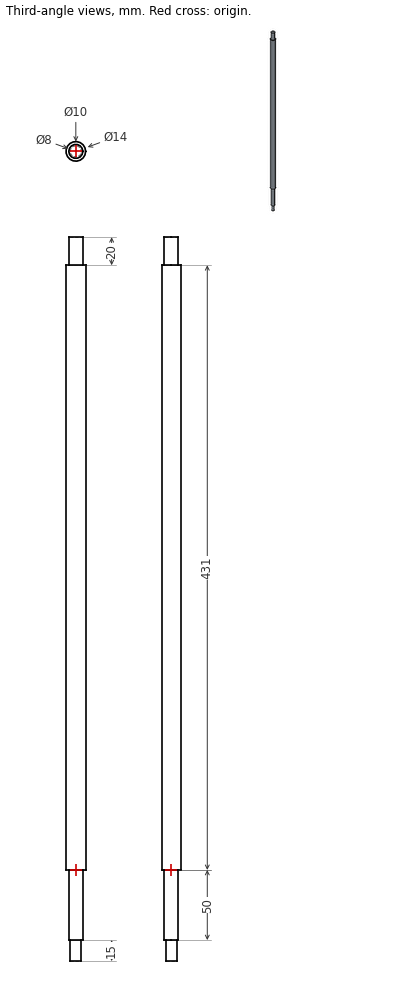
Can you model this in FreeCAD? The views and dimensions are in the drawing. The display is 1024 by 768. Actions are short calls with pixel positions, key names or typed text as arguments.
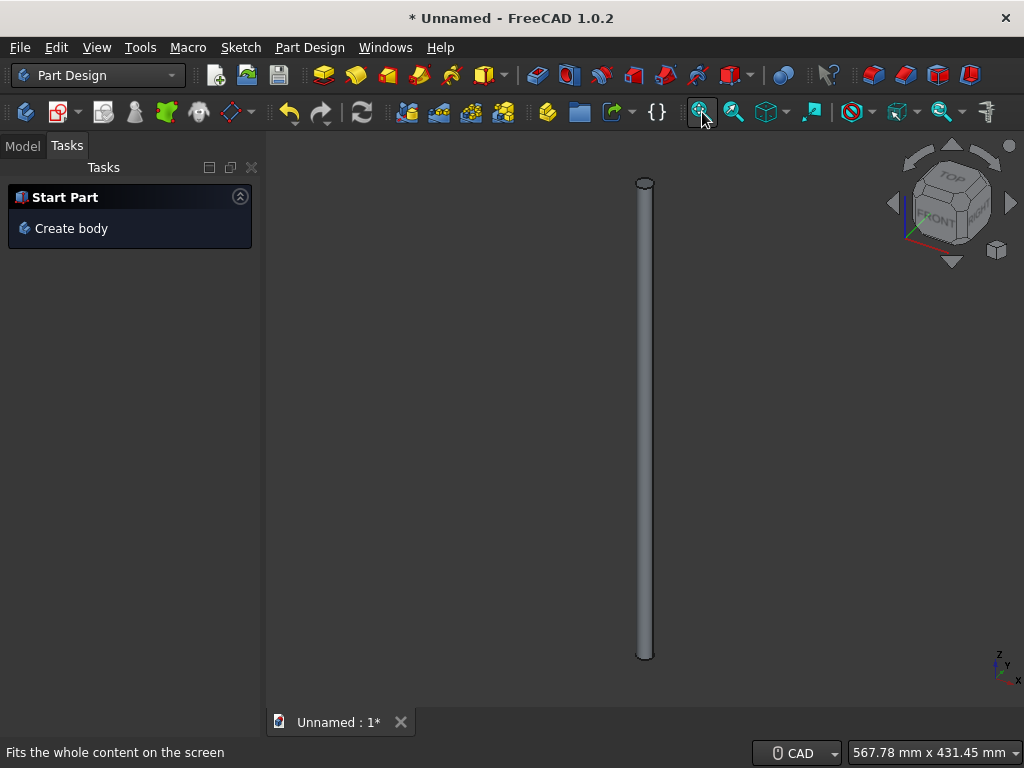
key(0)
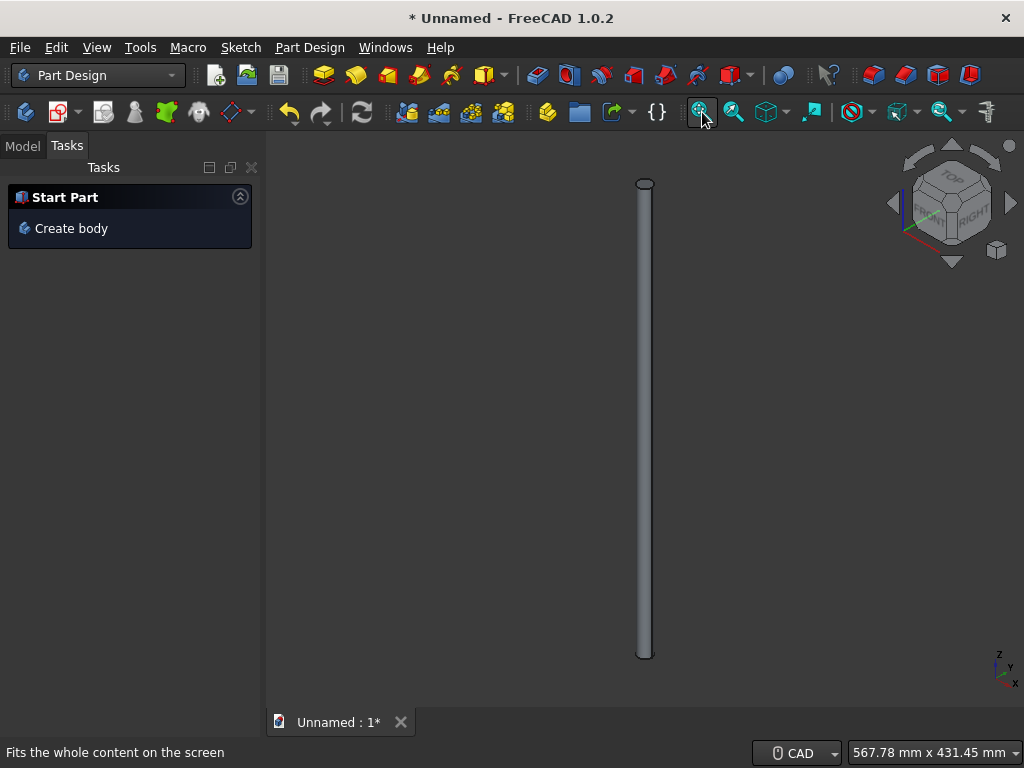
key(2)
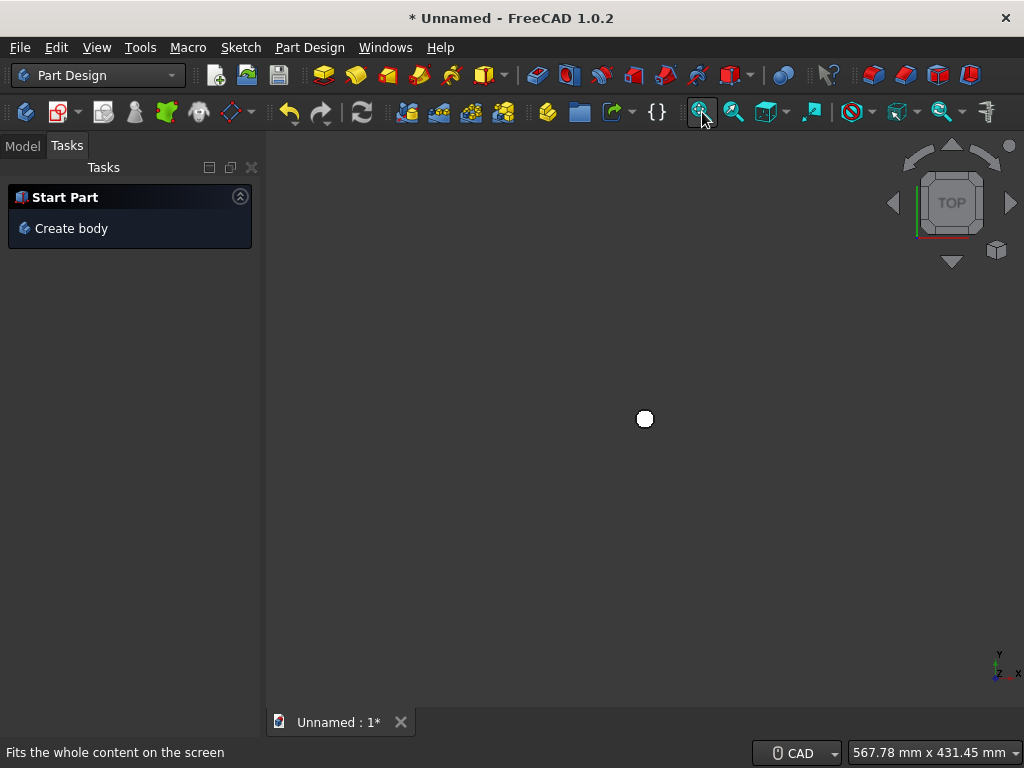
click(702, 112)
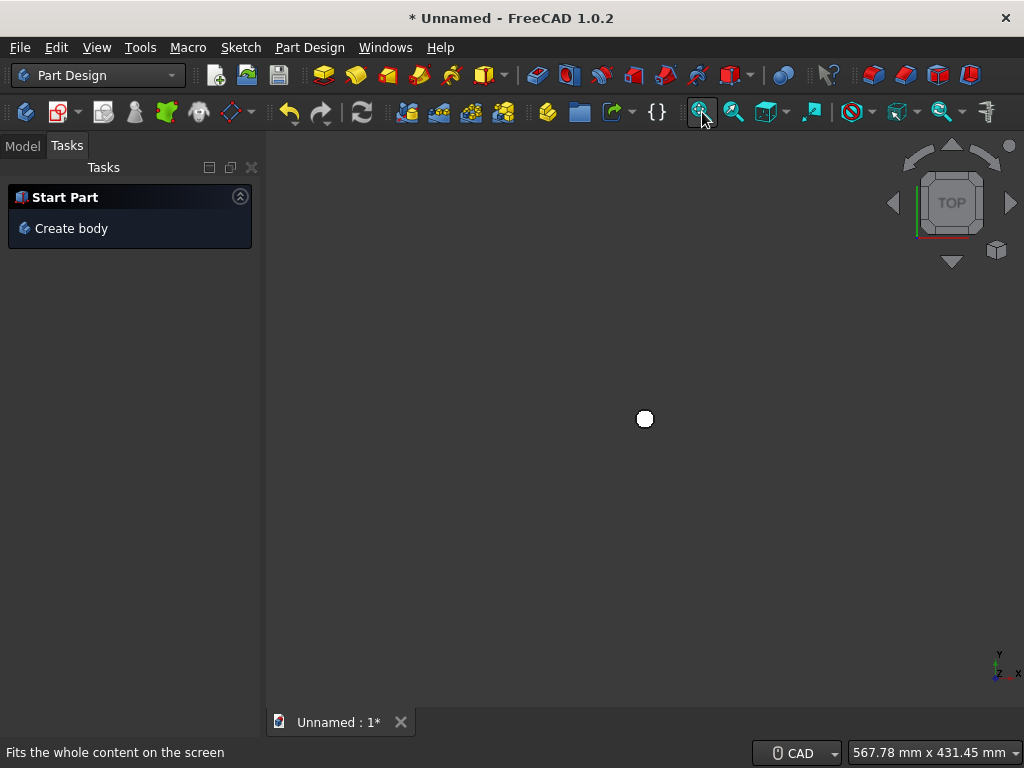
click(645, 418)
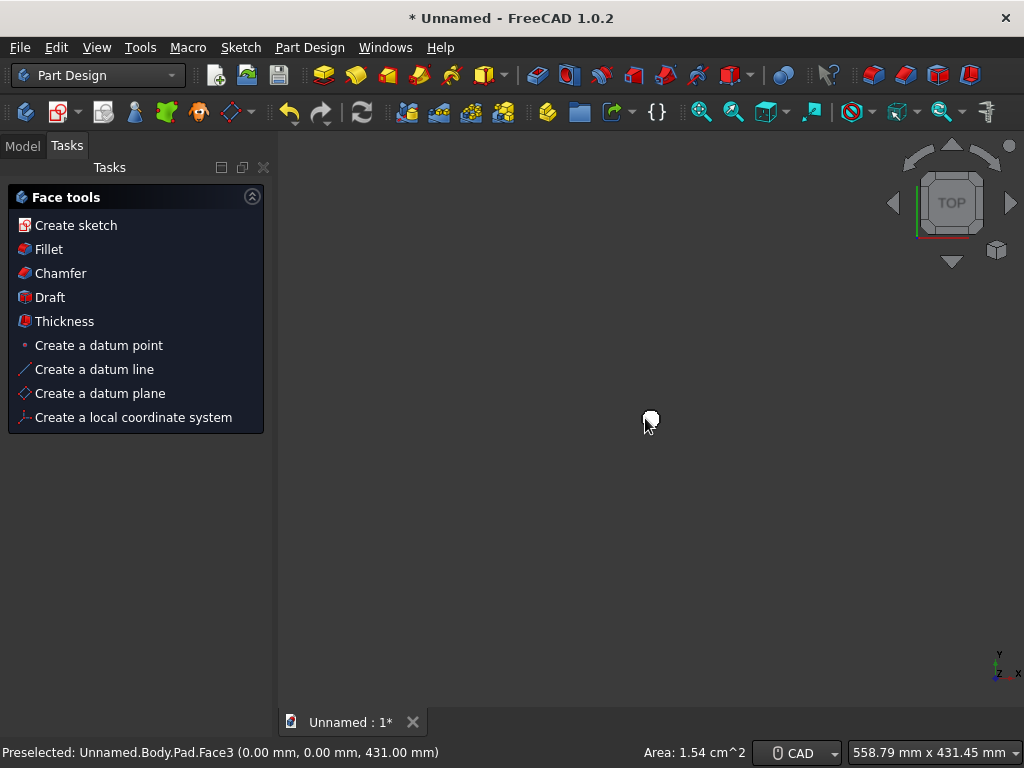
click(58, 112)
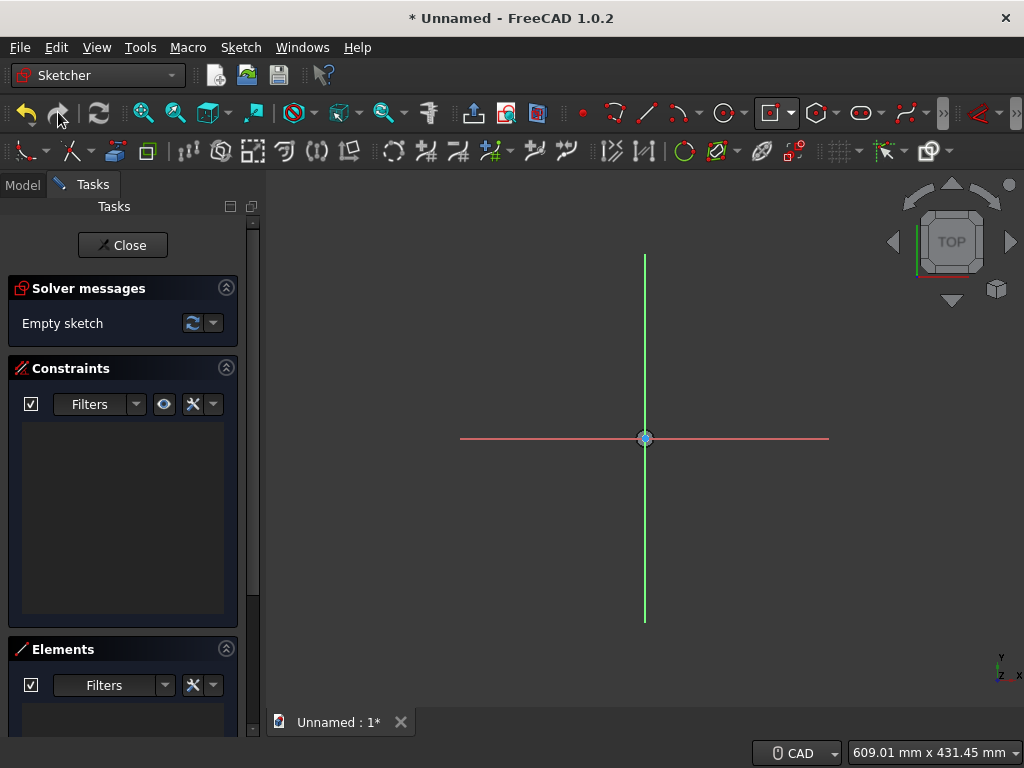
scroll(649, 438, up, 15)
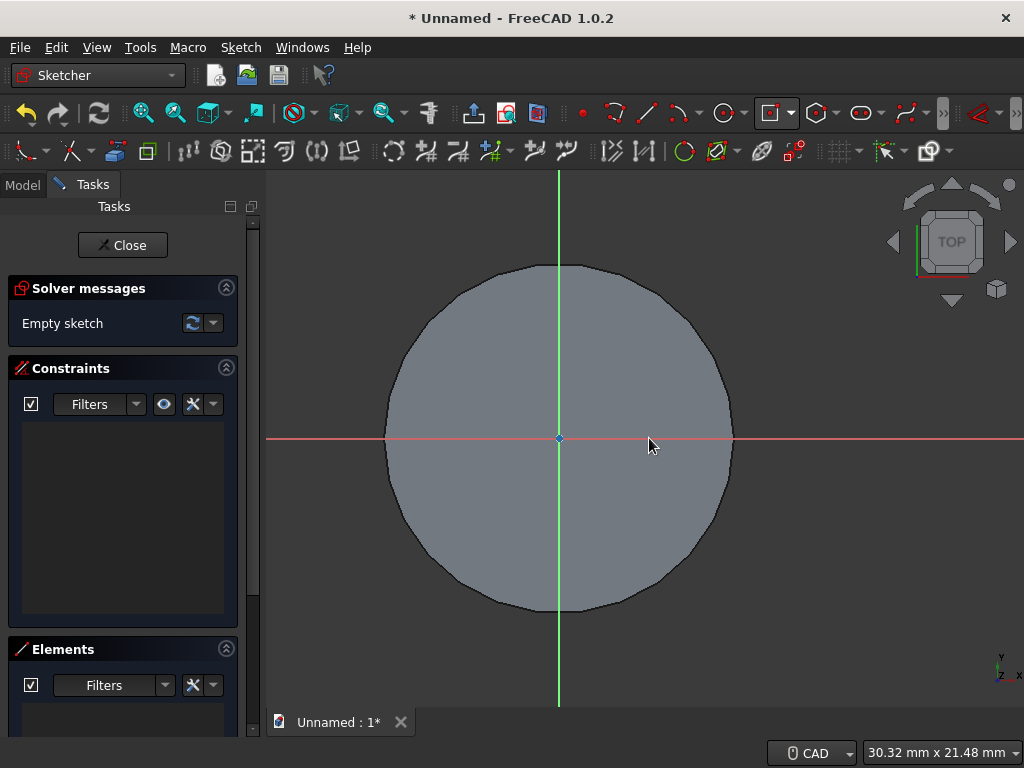
scroll(523, 439, up, 2)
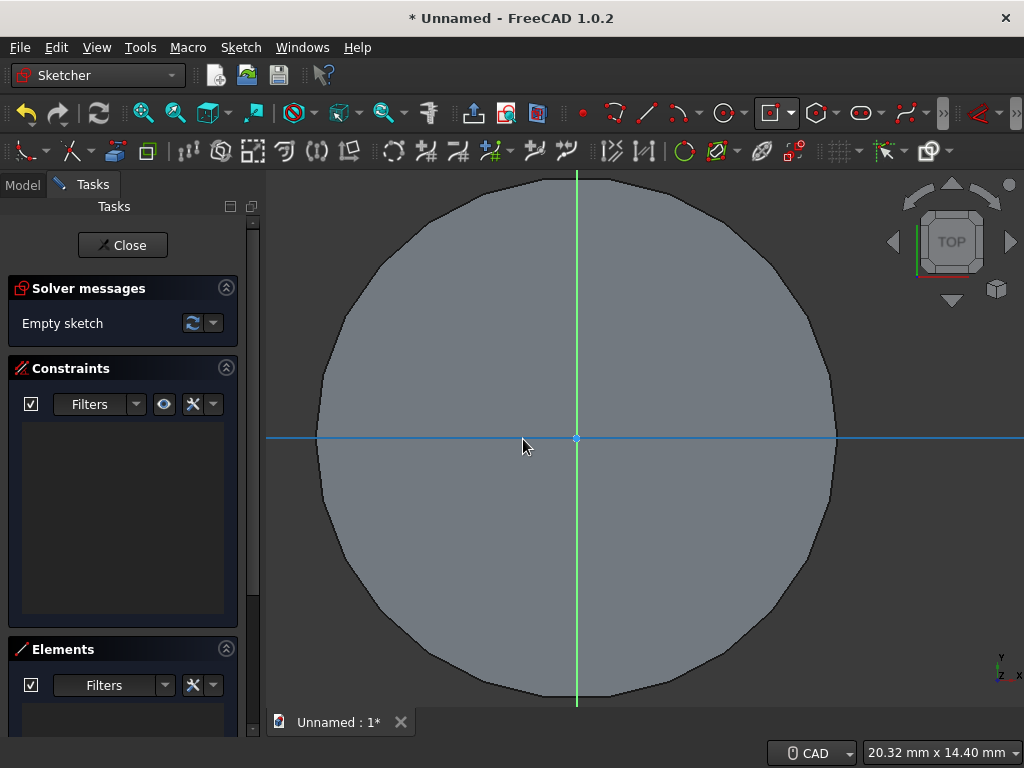
click(724, 114)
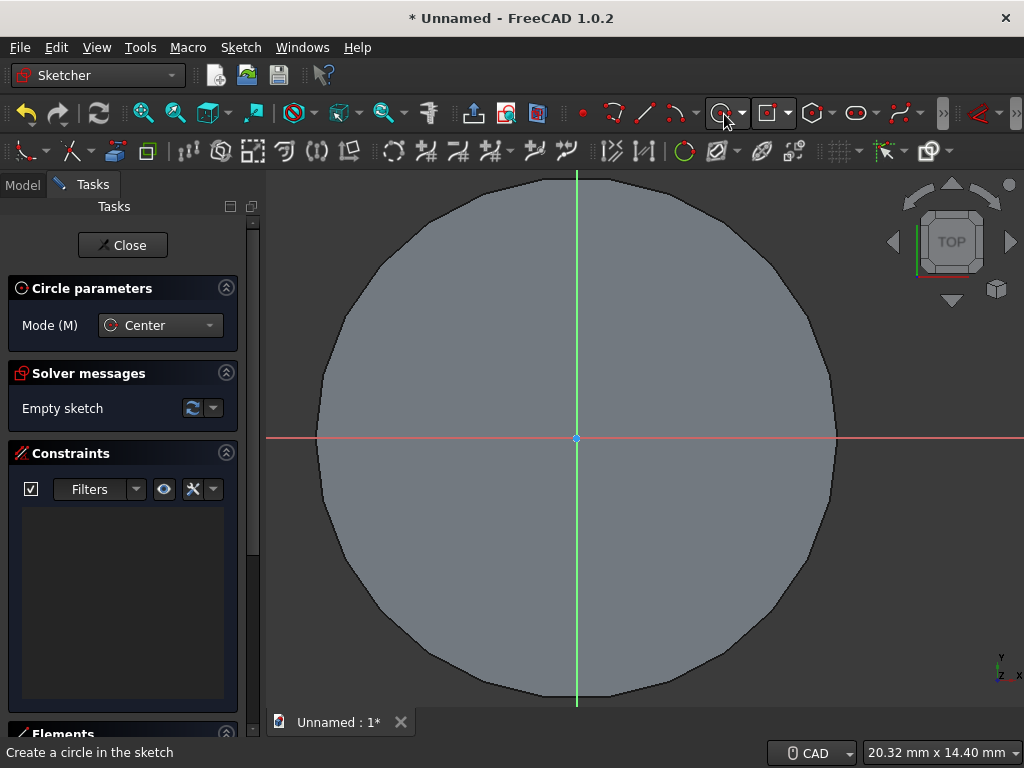
click(577, 438)
move(708, 306)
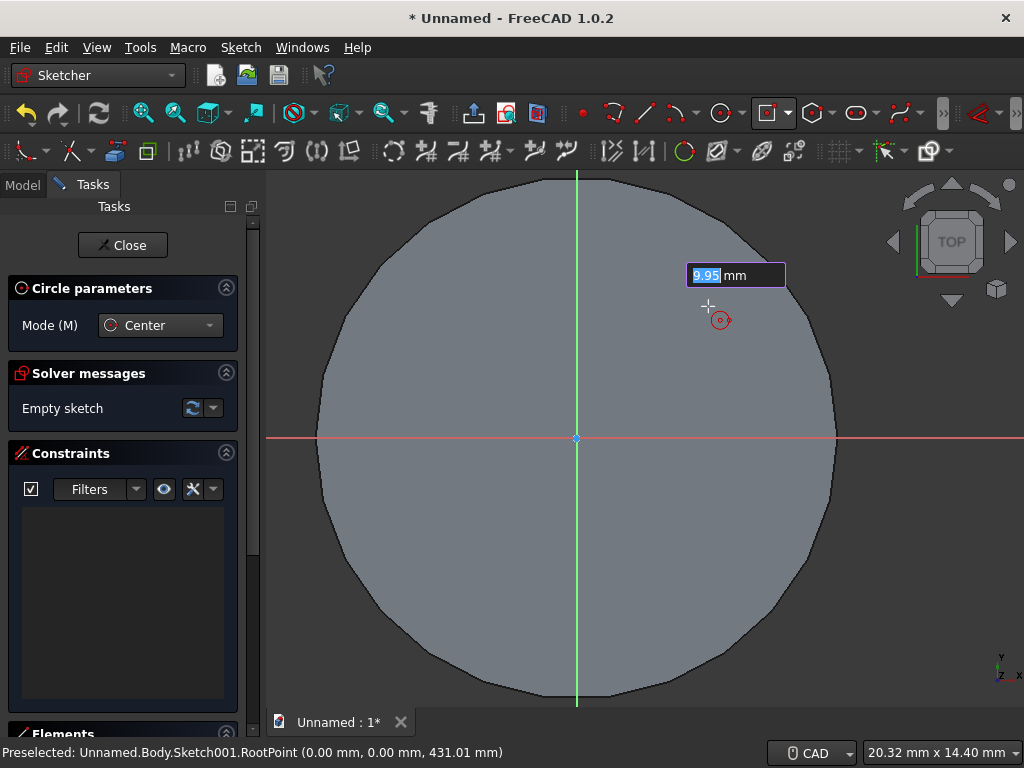
text(10)
key(Return)
key(Escape)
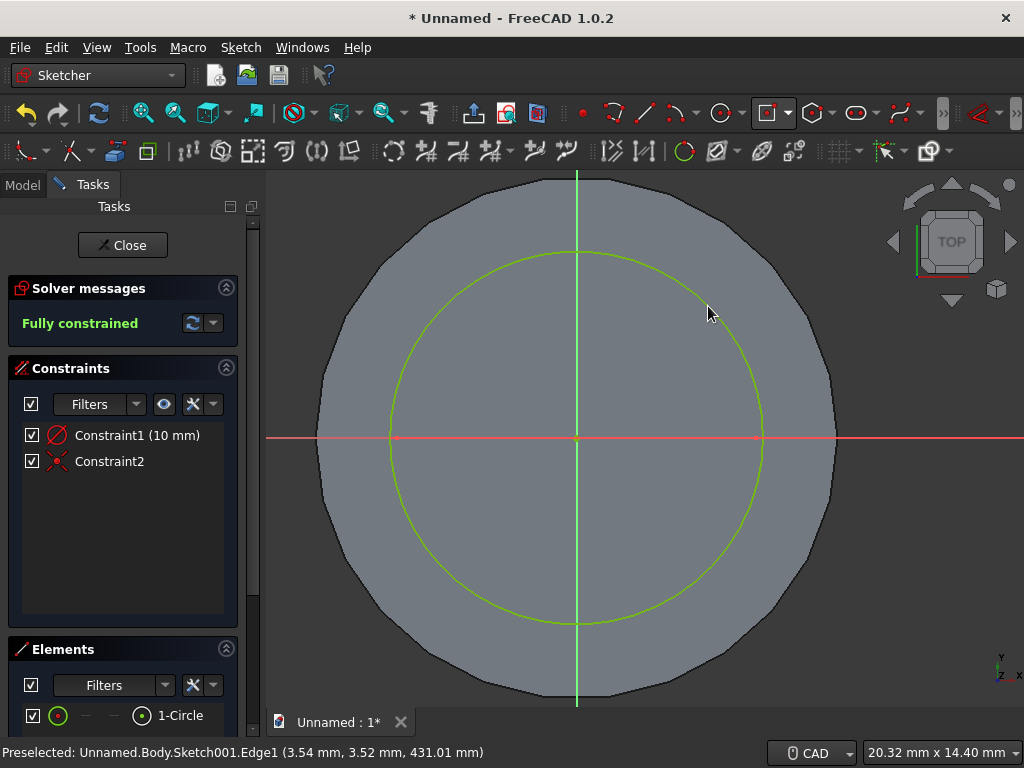
click(123, 245)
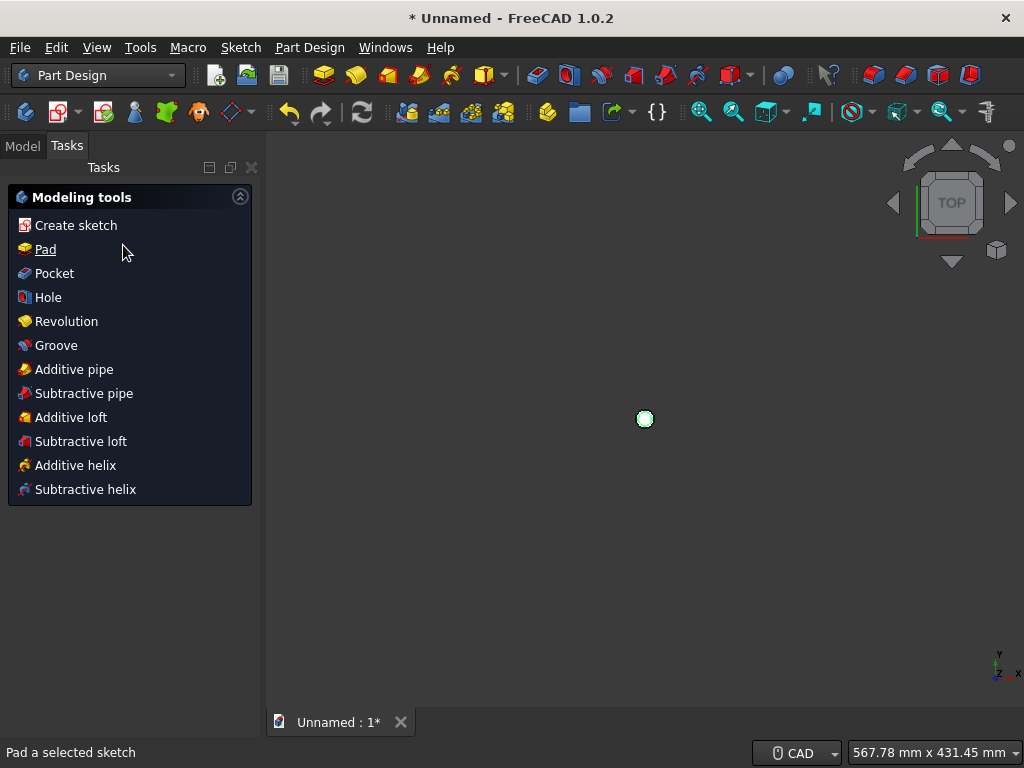
click(324, 76)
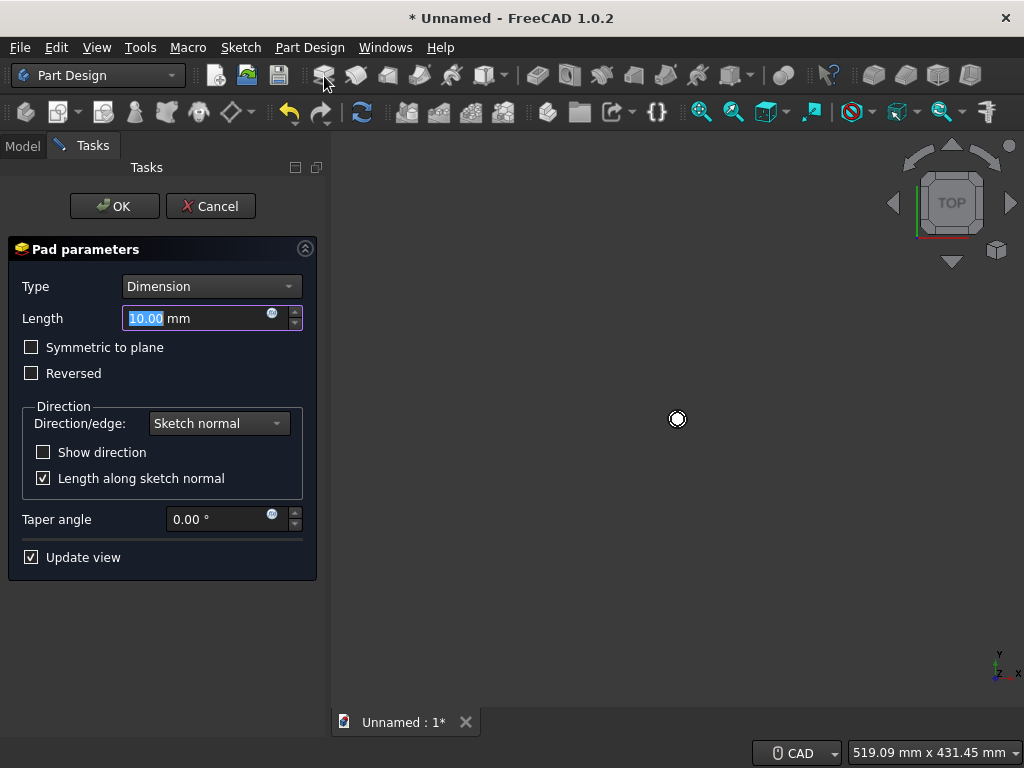
text(20)
key(Tab)